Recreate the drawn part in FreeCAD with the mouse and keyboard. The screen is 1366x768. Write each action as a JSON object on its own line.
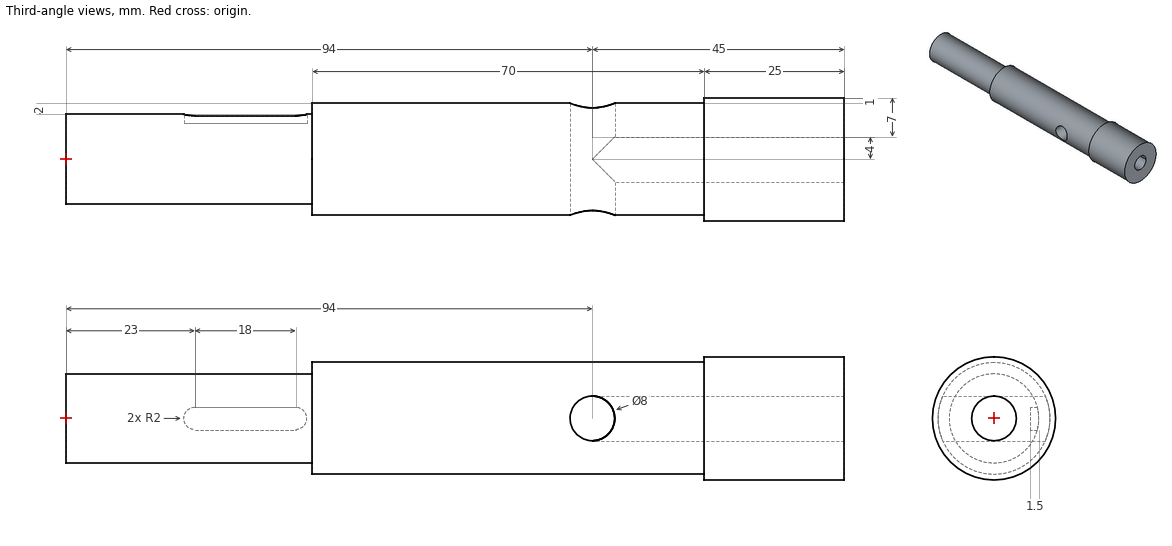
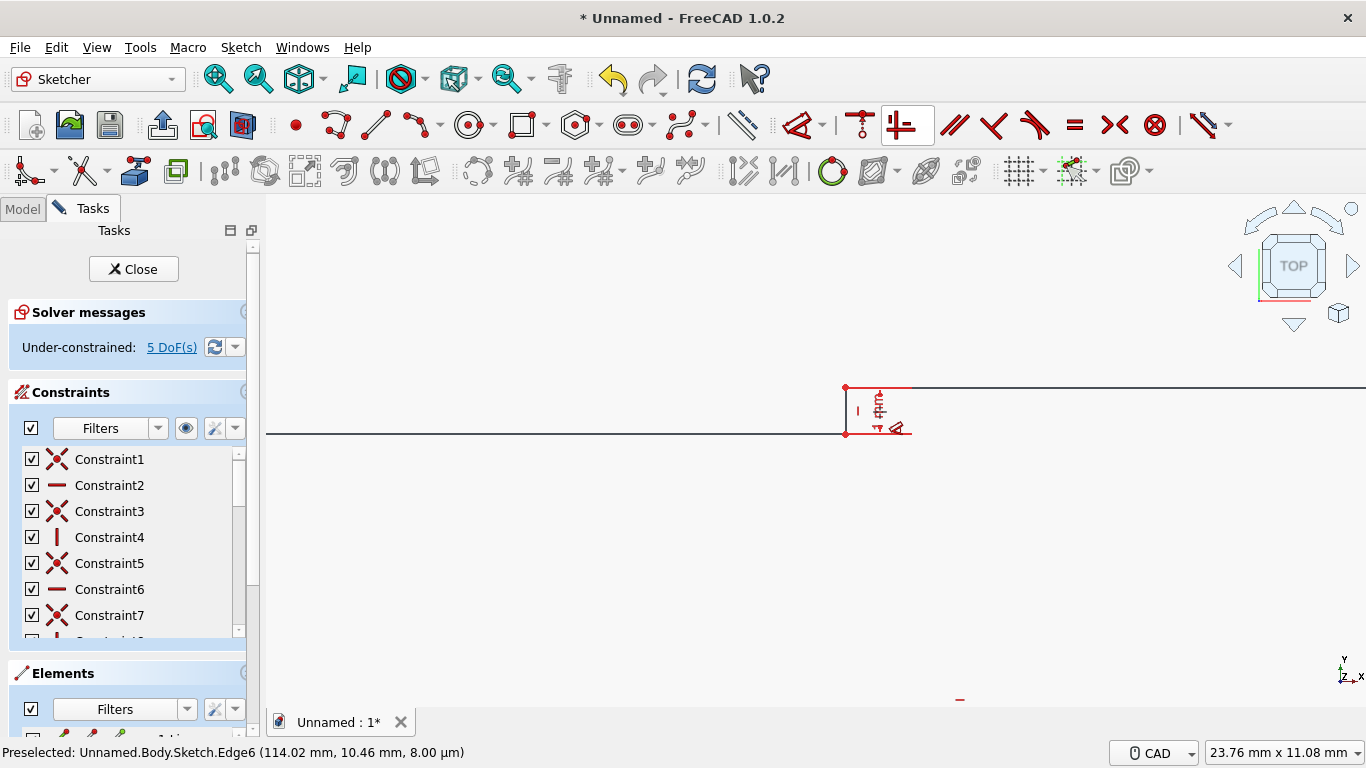
{"action": "scroll", "coordinate": [943, 431], "scroll_direction": "down", "scroll_amount": 12}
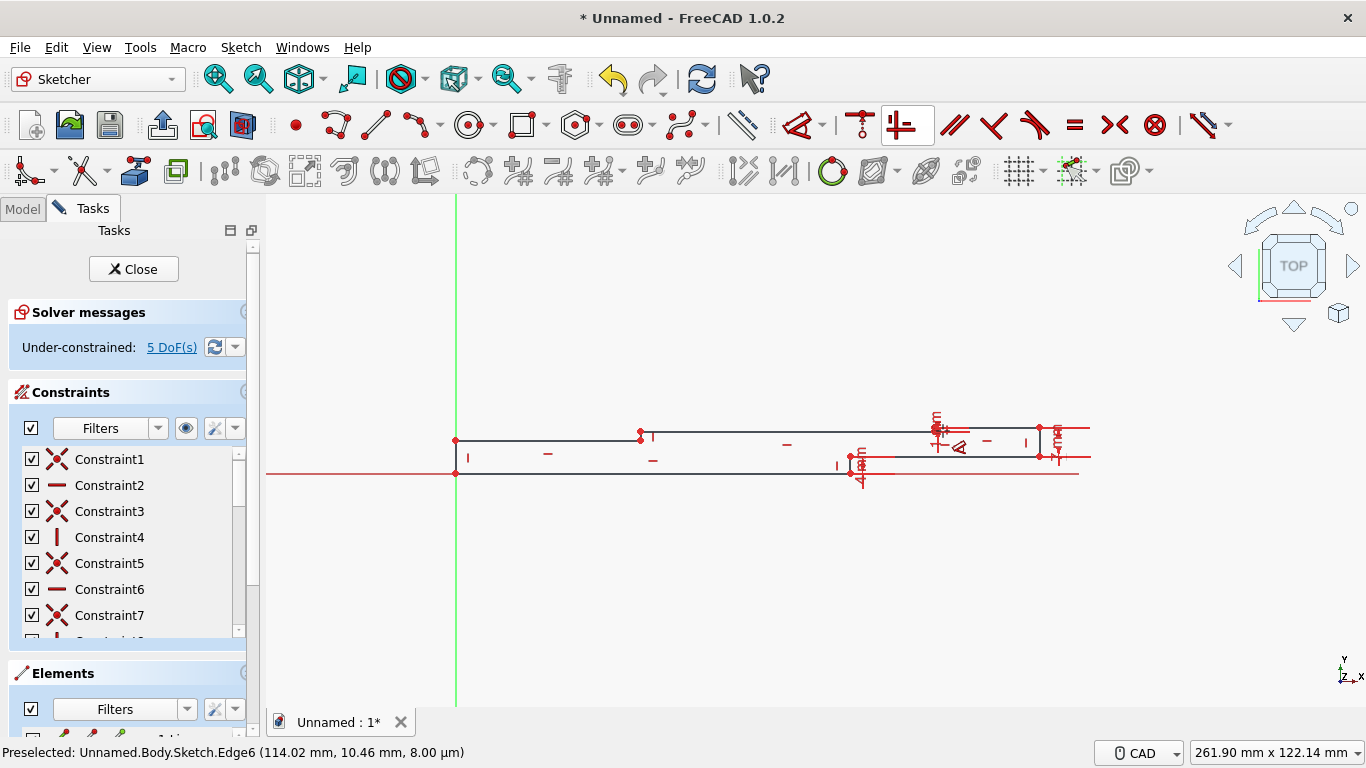
{"action": "scroll", "coordinate": [641, 434], "scroll_direction": "up", "scroll_amount": 9}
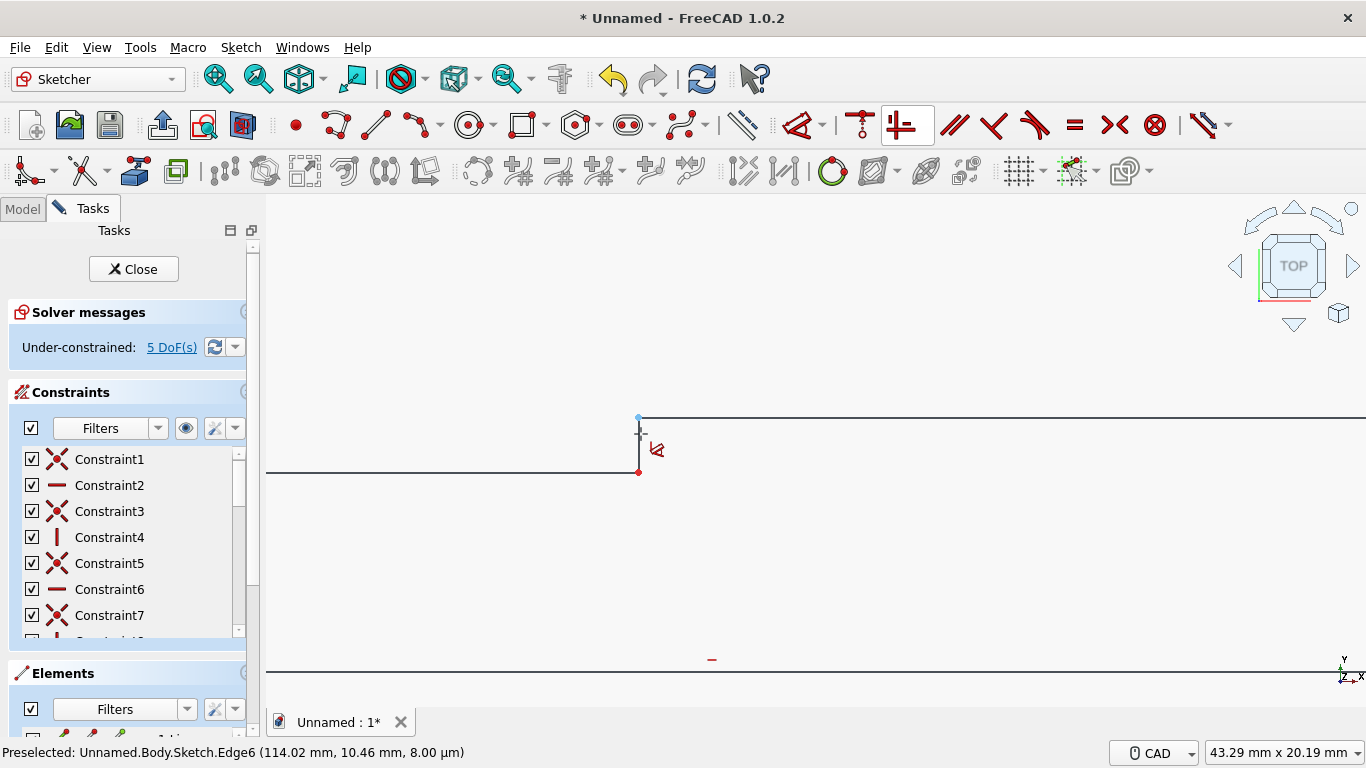
{"action": "left_click", "coordinate": [639, 434]}
{"action": "left_click", "coordinate": [605, 445]}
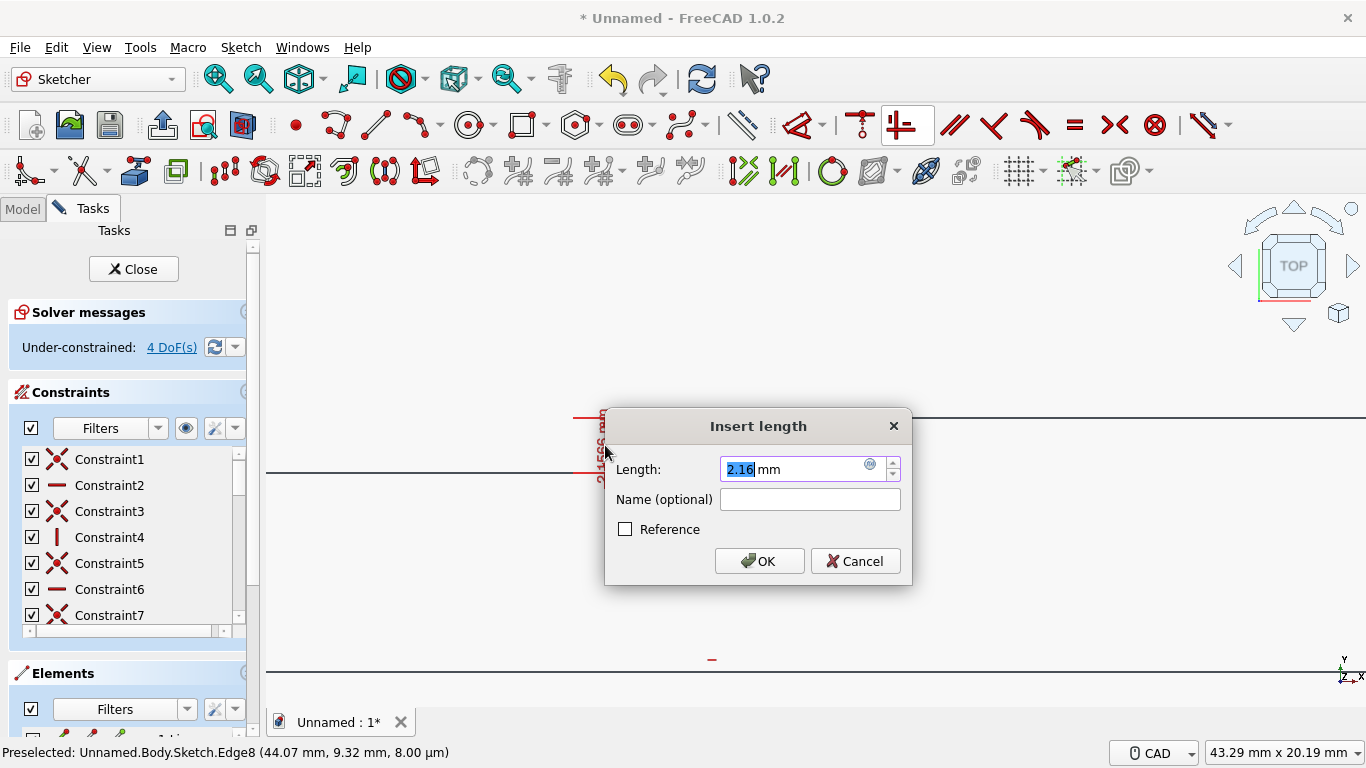
{"action": "type", "text": "2"}
{"action": "key", "text": "Return"}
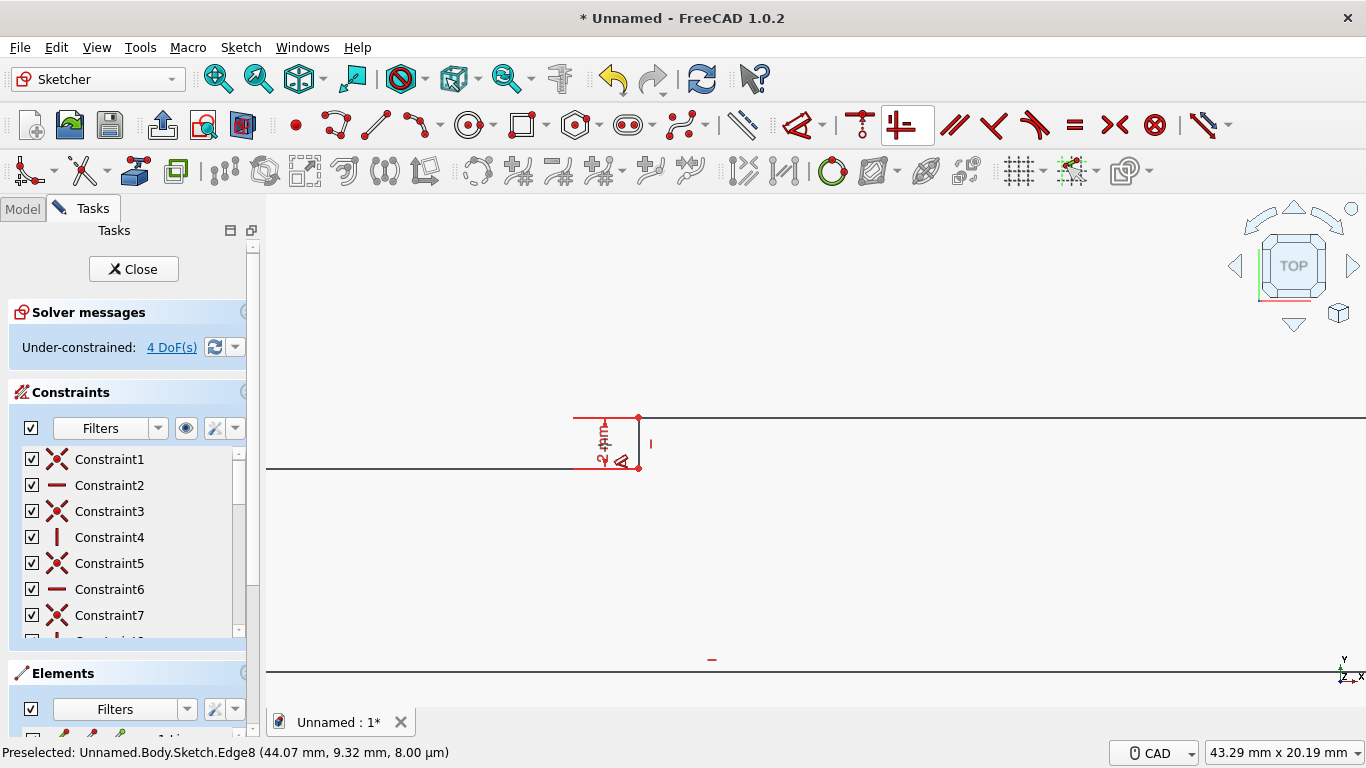
{"action": "scroll", "coordinate": [641, 434], "scroll_direction": "down", "scroll_amount": 9}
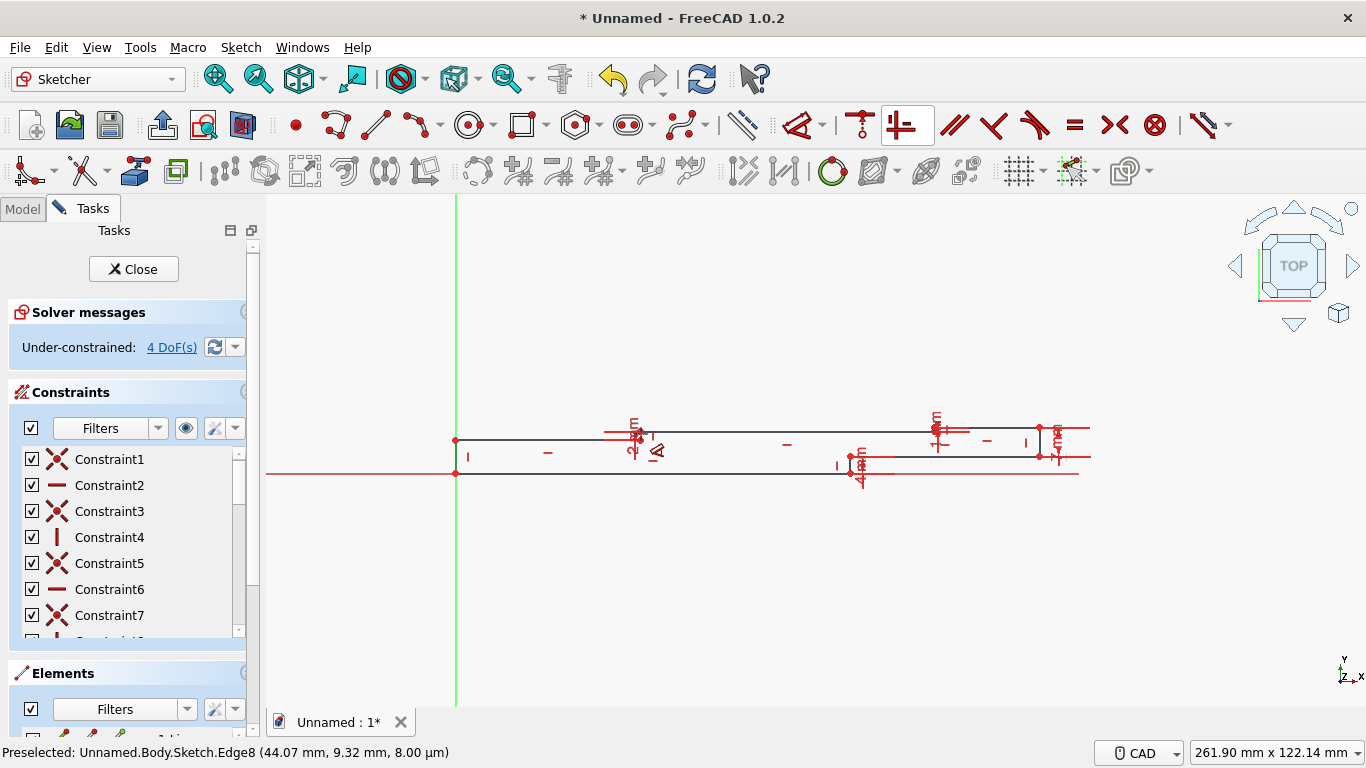
{"action": "left_click", "coordinate": [732, 474]}
{"action": "left_click", "coordinate": [653, 508]}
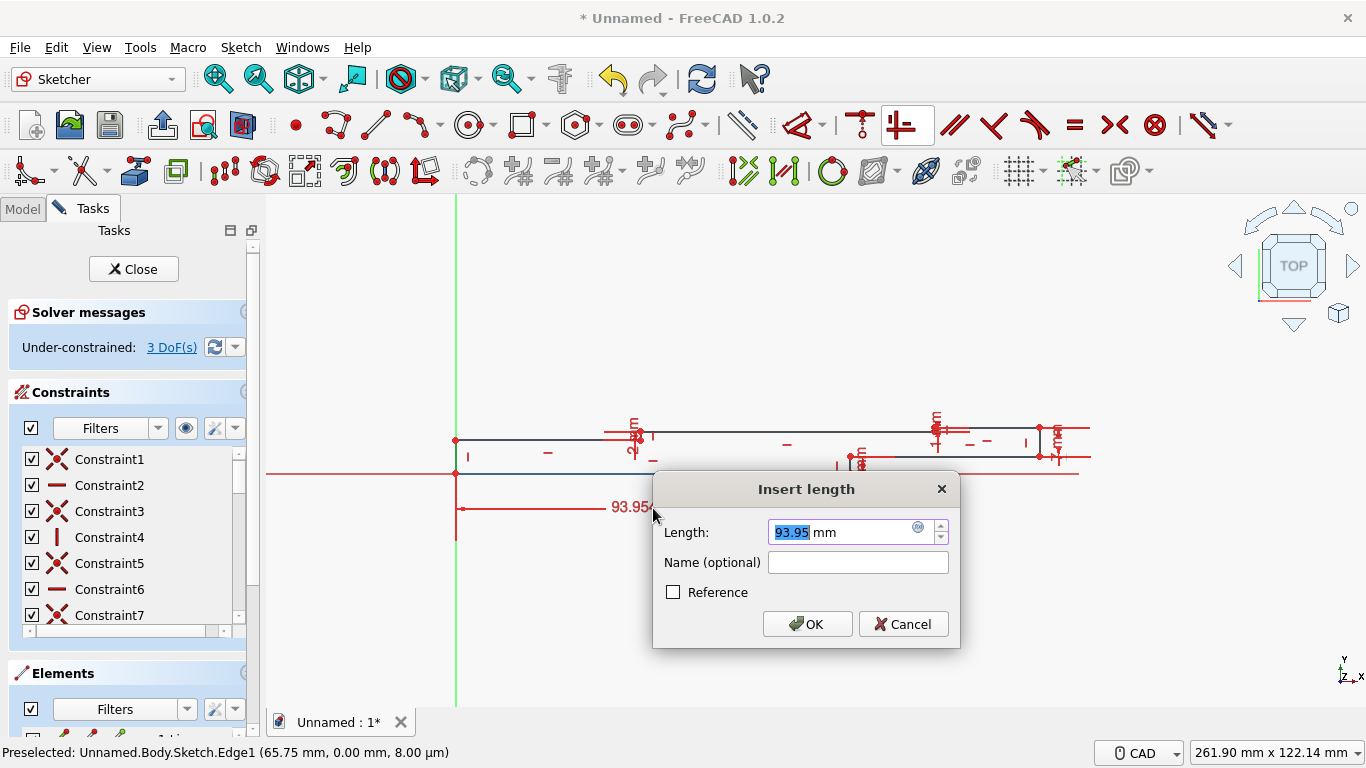
{"action": "type", "text": "94"}
{"action": "key", "text": "Return"}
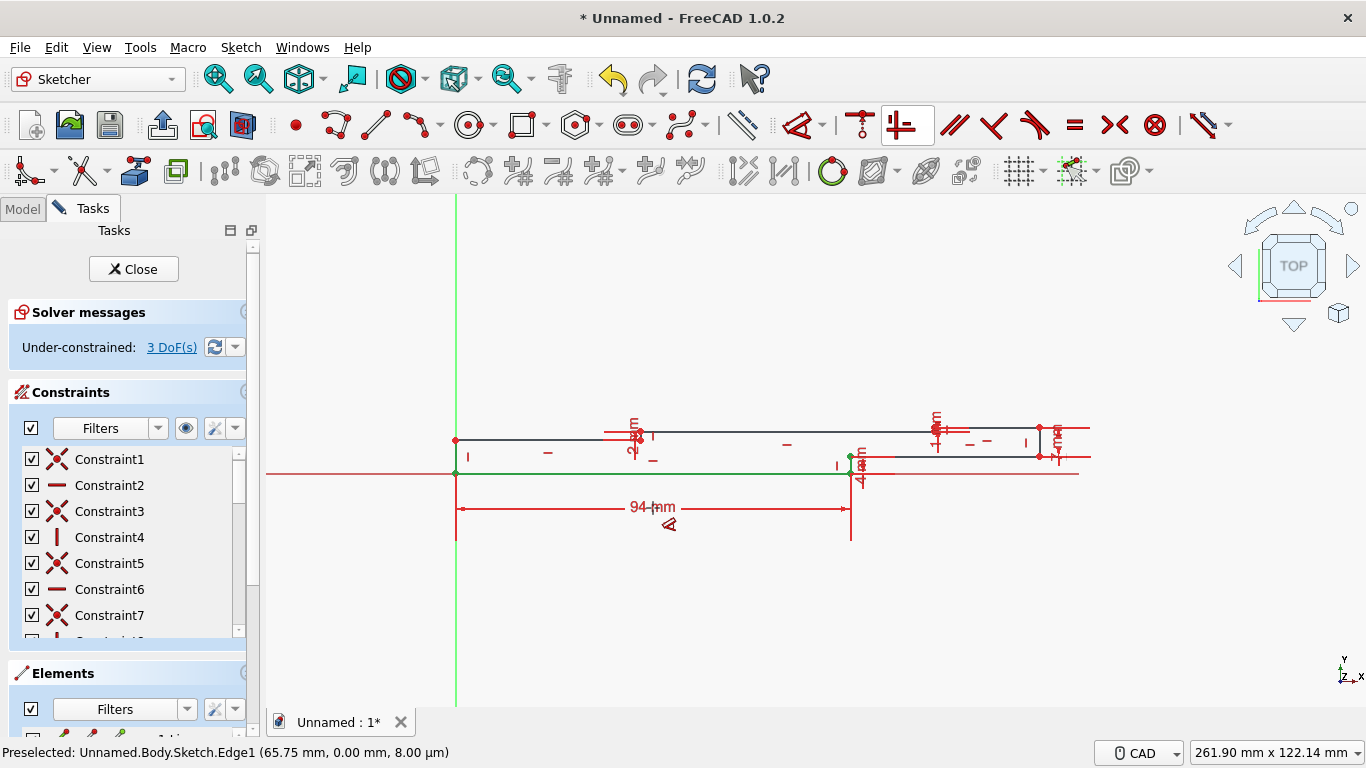
{"action": "left_click", "coordinate": [907, 457]}
{"action": "left_click", "coordinate": [945, 491]}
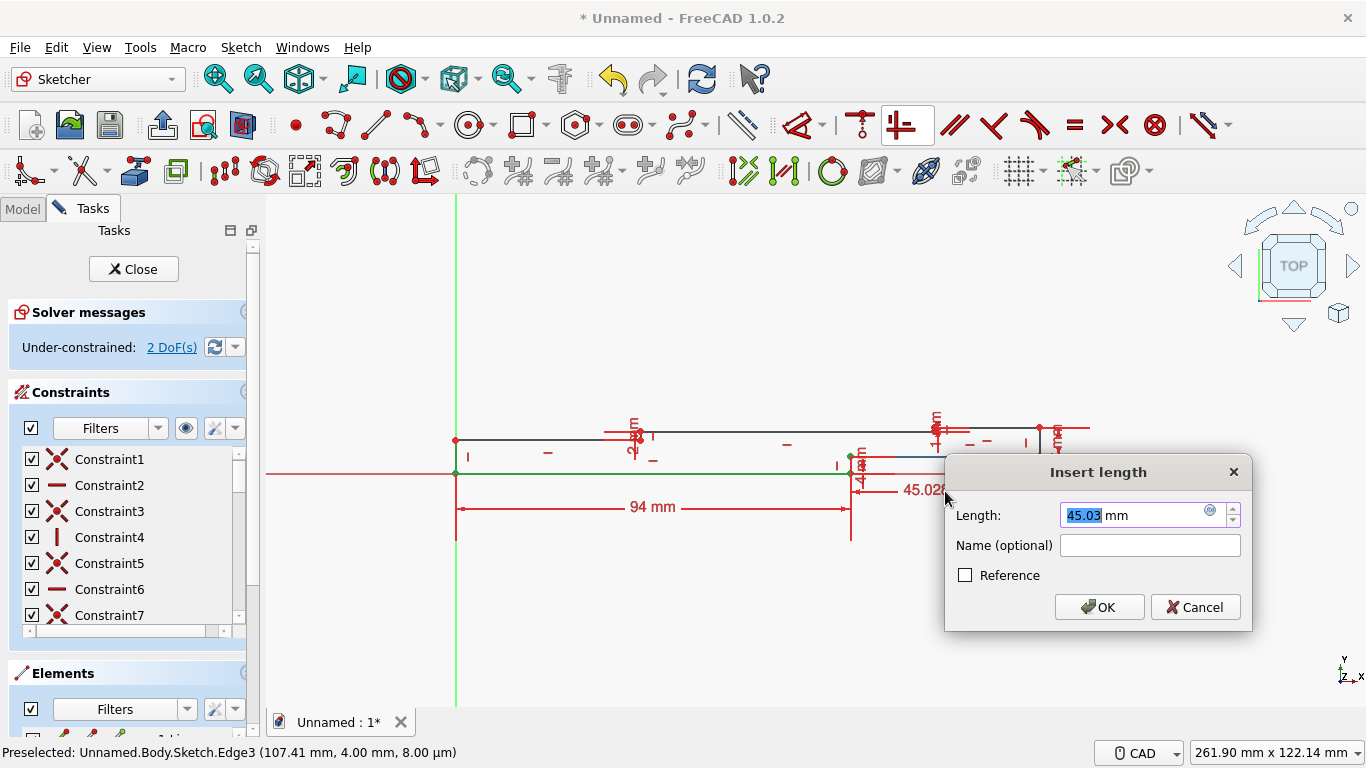
{"action": "type", "text": "45"}
{"action": "key", "text": "Return"}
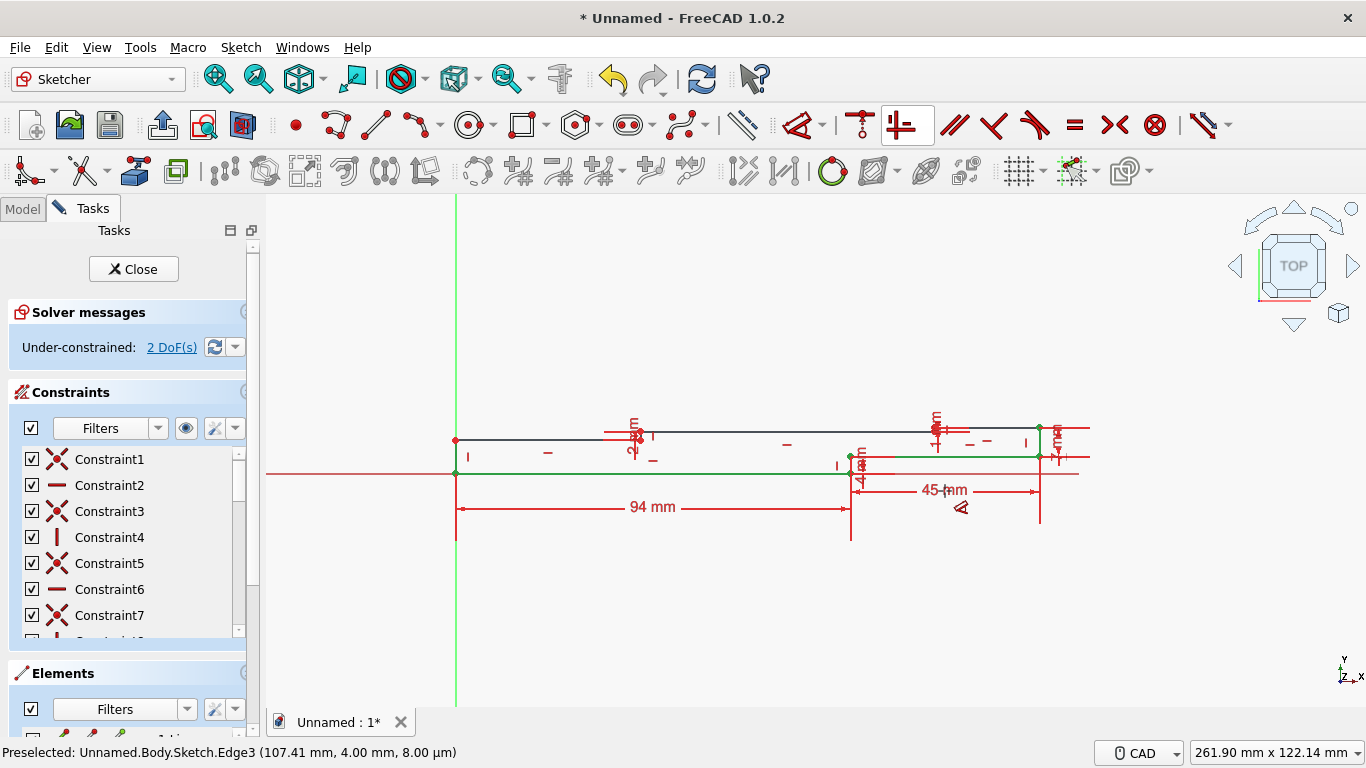
{"action": "left_click", "coordinate": [1008, 428]}
{"action": "left_click", "coordinate": [987, 394]}